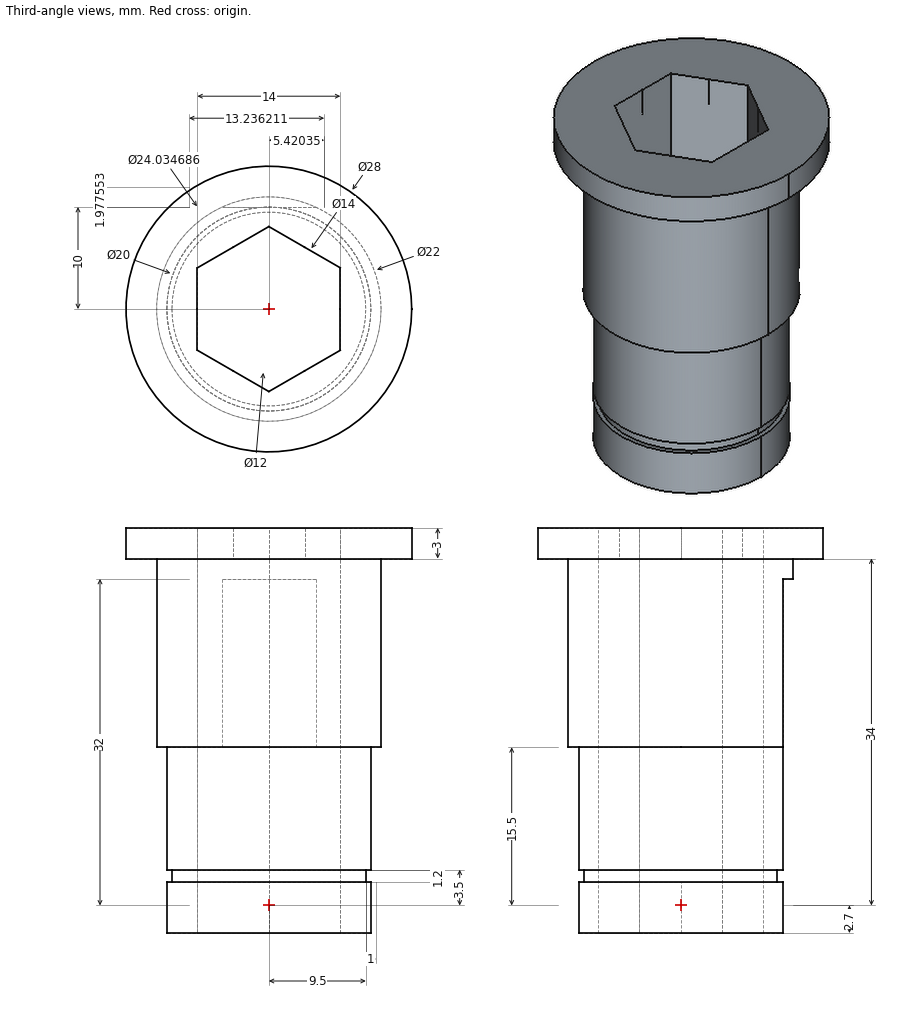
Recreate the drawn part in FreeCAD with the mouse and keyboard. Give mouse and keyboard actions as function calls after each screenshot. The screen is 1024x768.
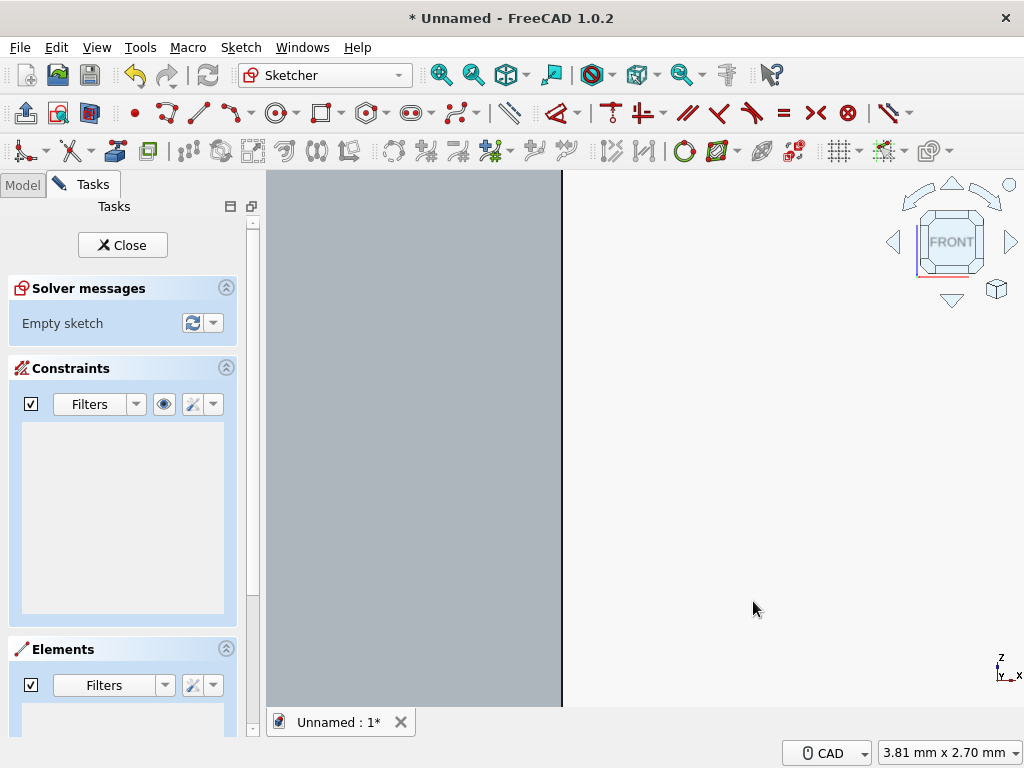
scroll(532, 402, up, 2)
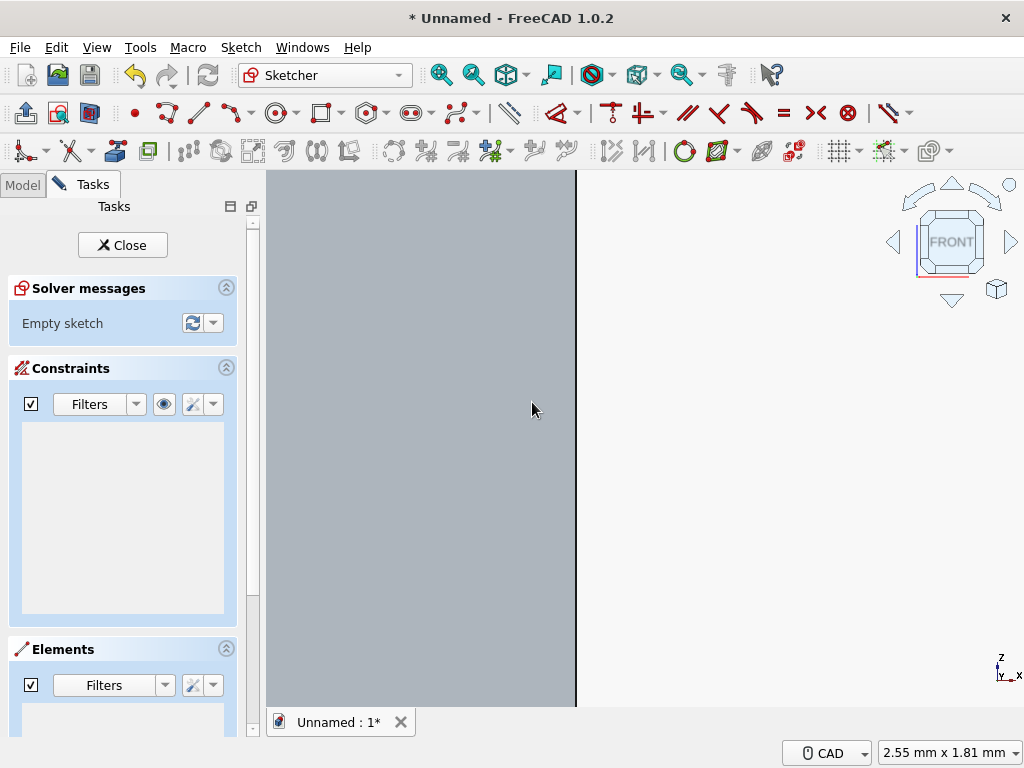
click(322, 114)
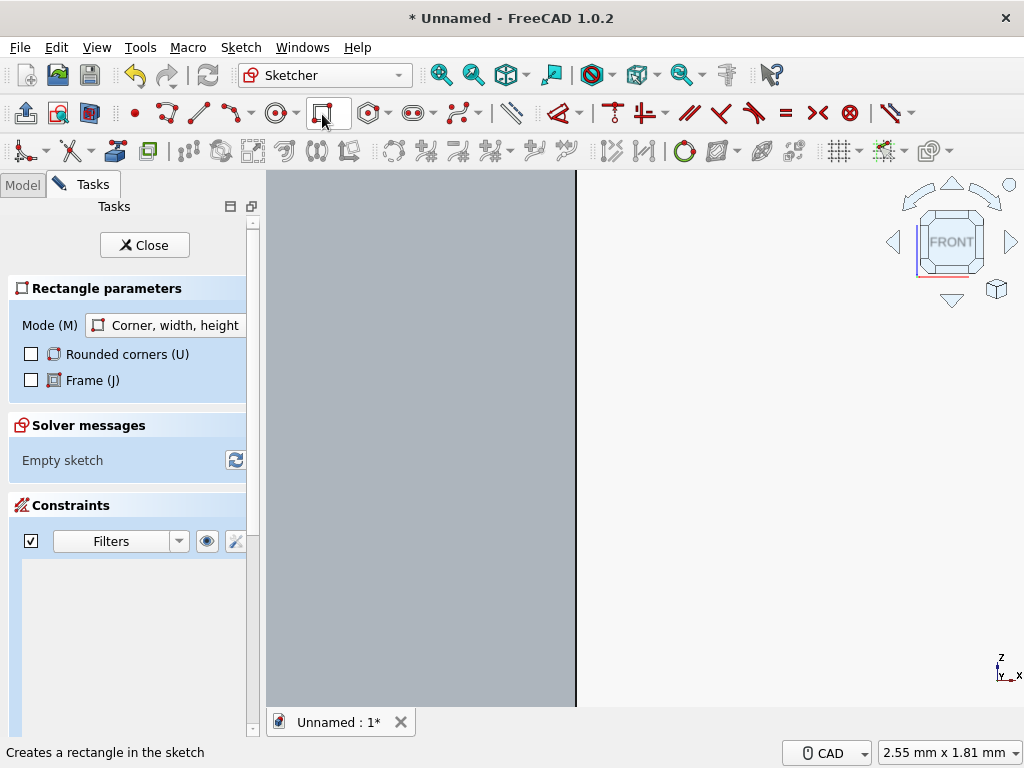
click(428, 260)
click(725, 617)
key(Escape)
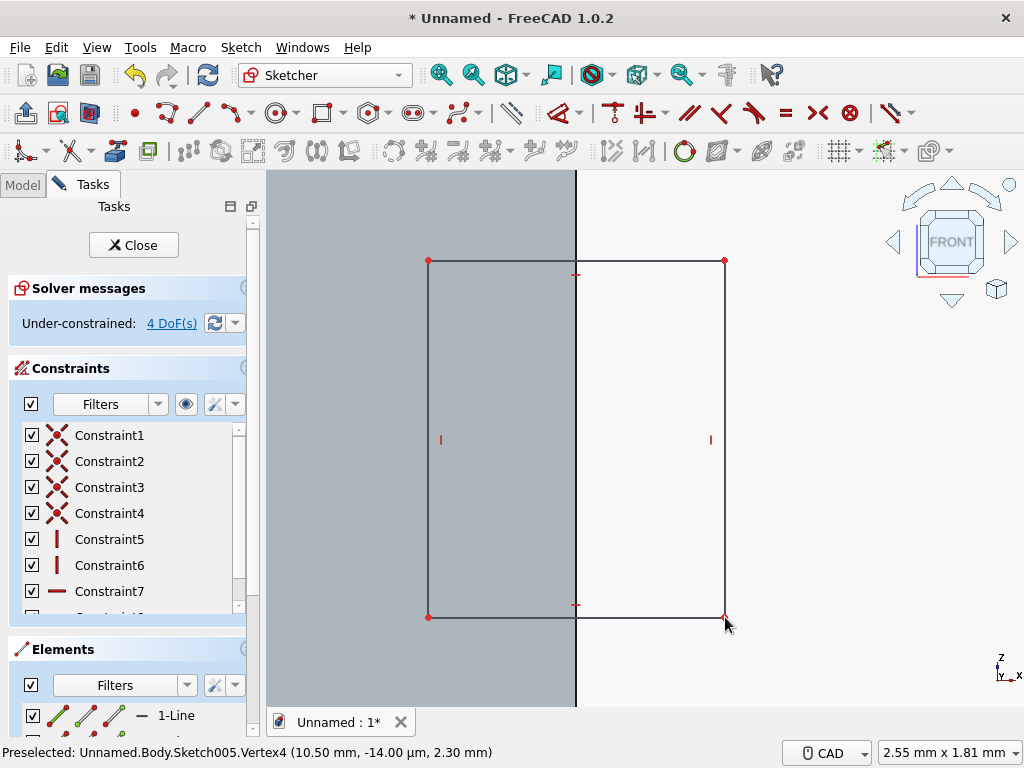
click(558, 114)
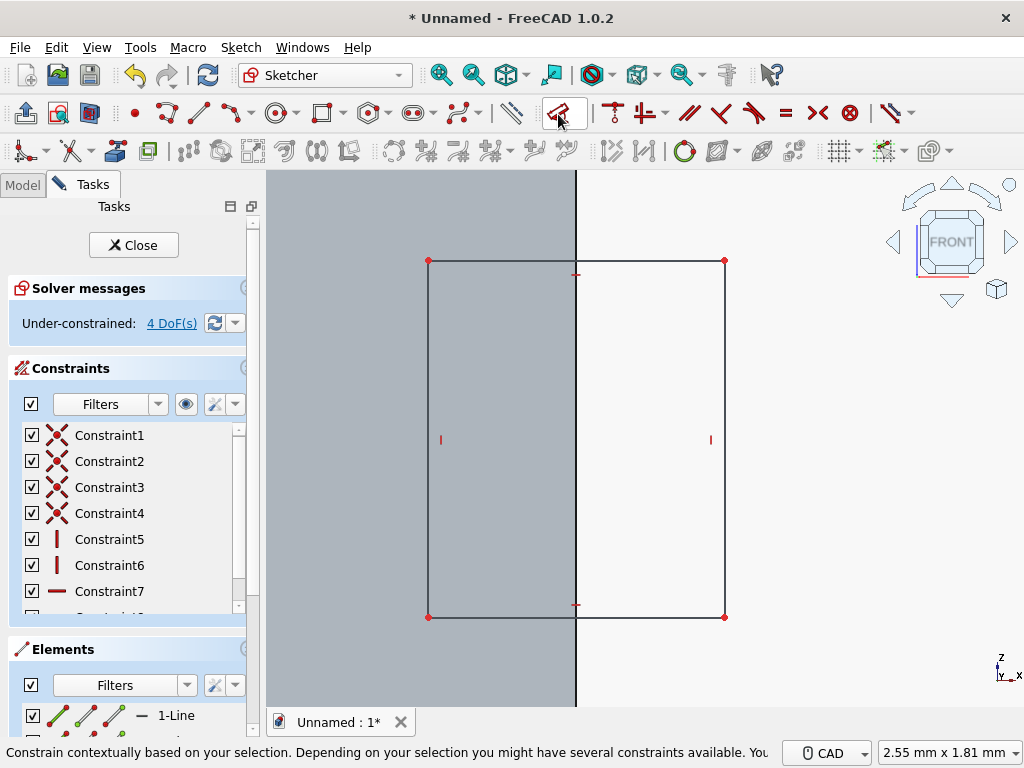
click(517, 618)
click(576, 652)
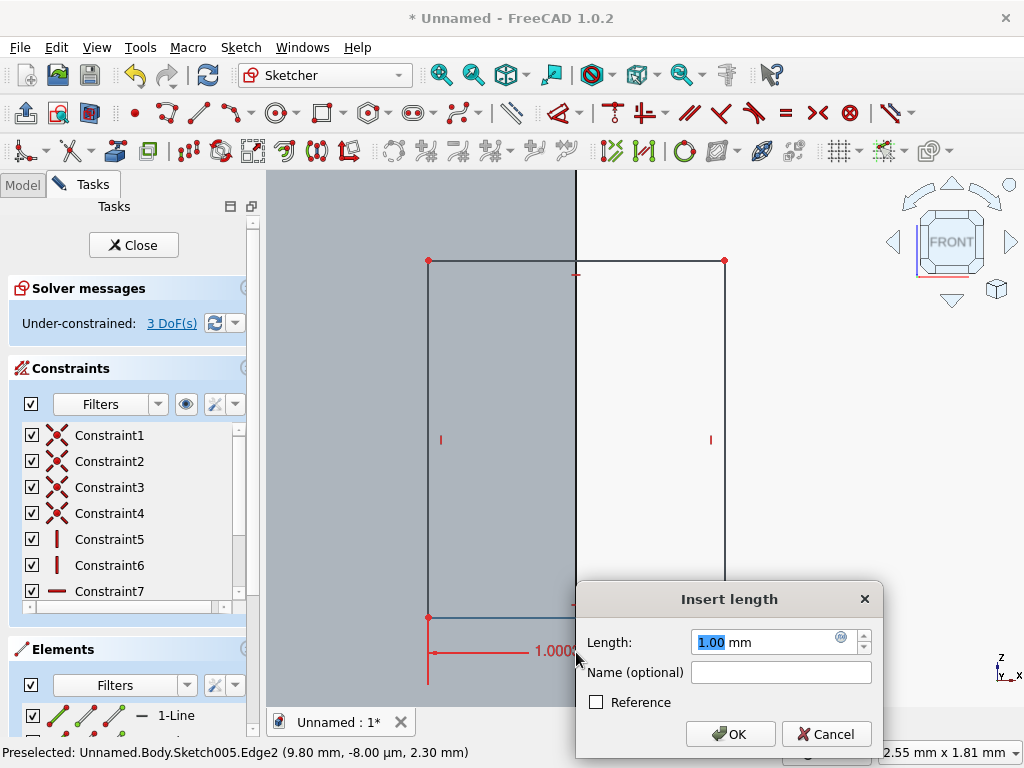
text(1)
key(Return)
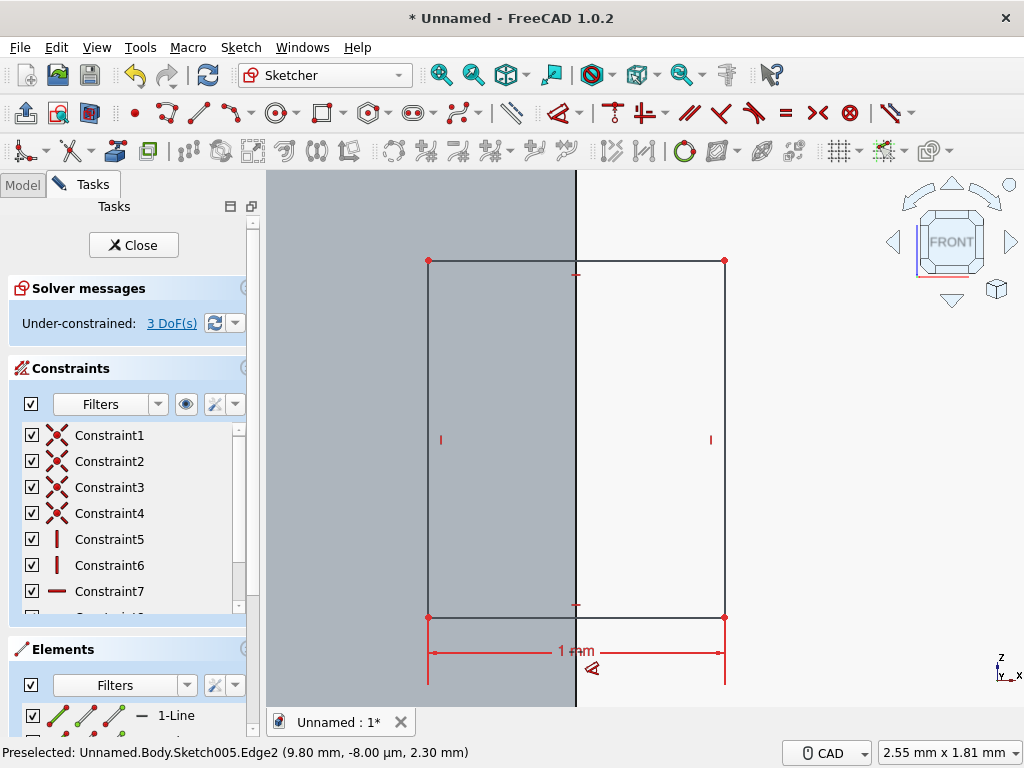
click(428, 368)
click(394, 440)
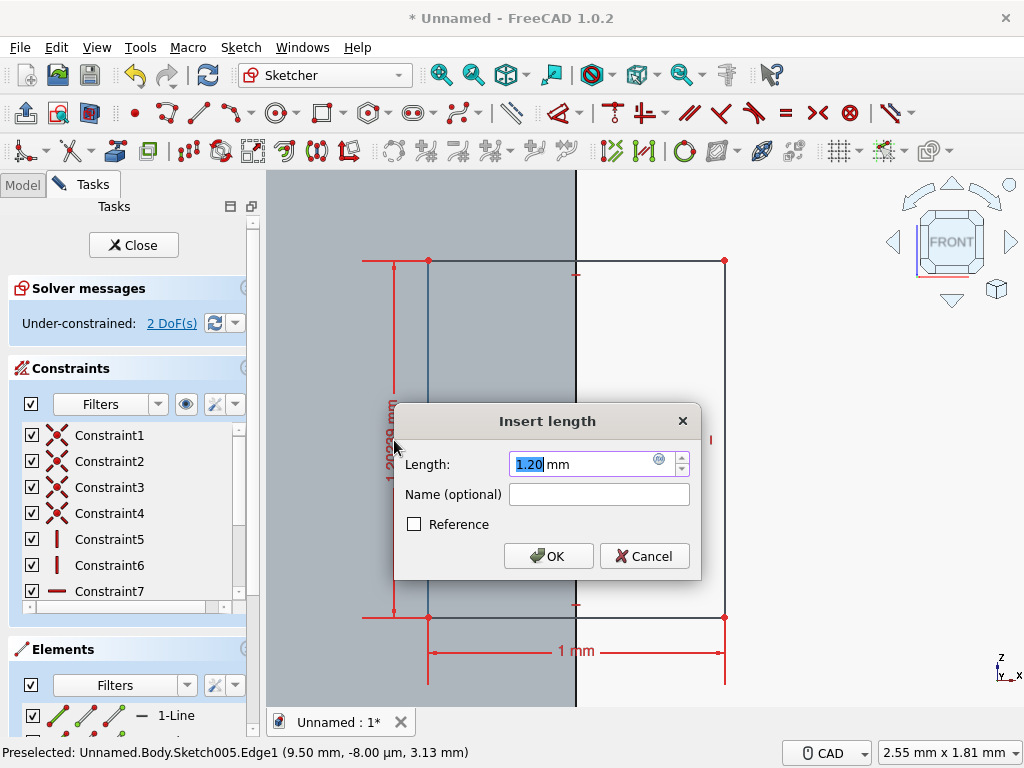
text(1.2)
key(Return)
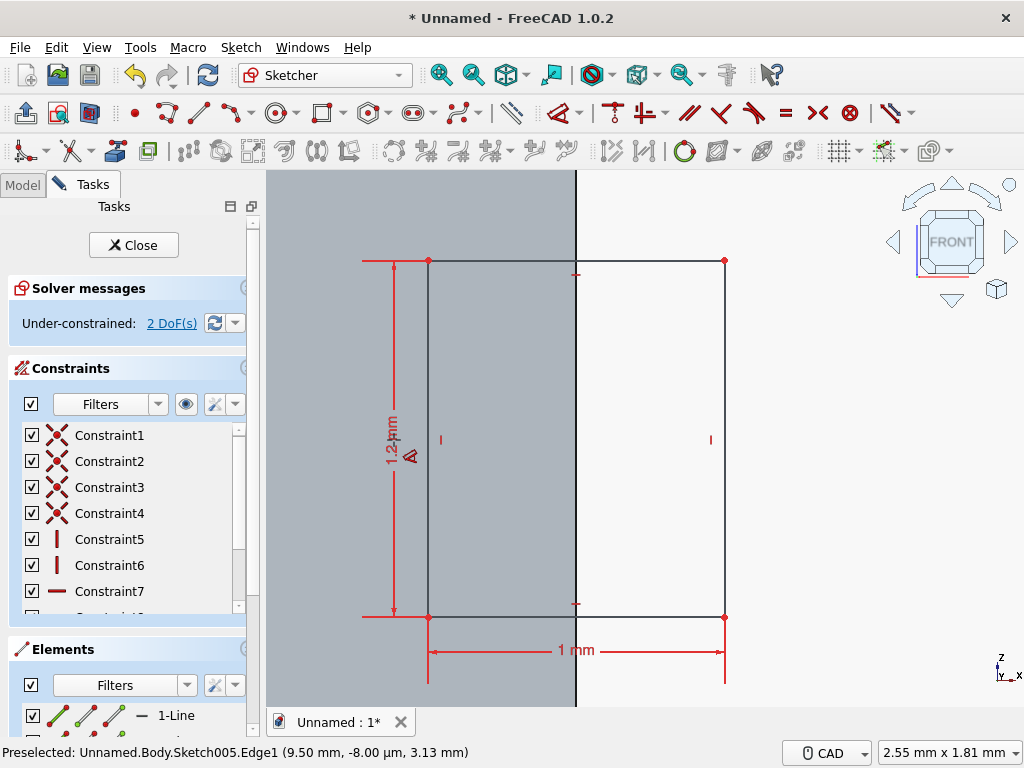
click(428, 261)
click(361, 227)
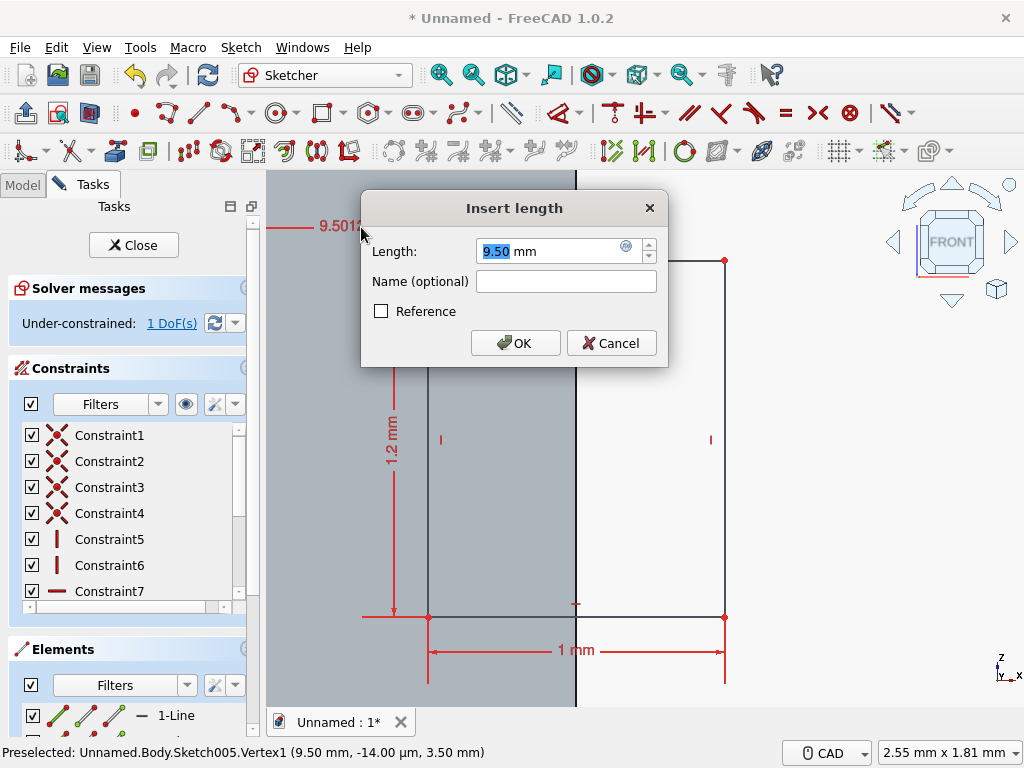
text(9.5)
key(Return)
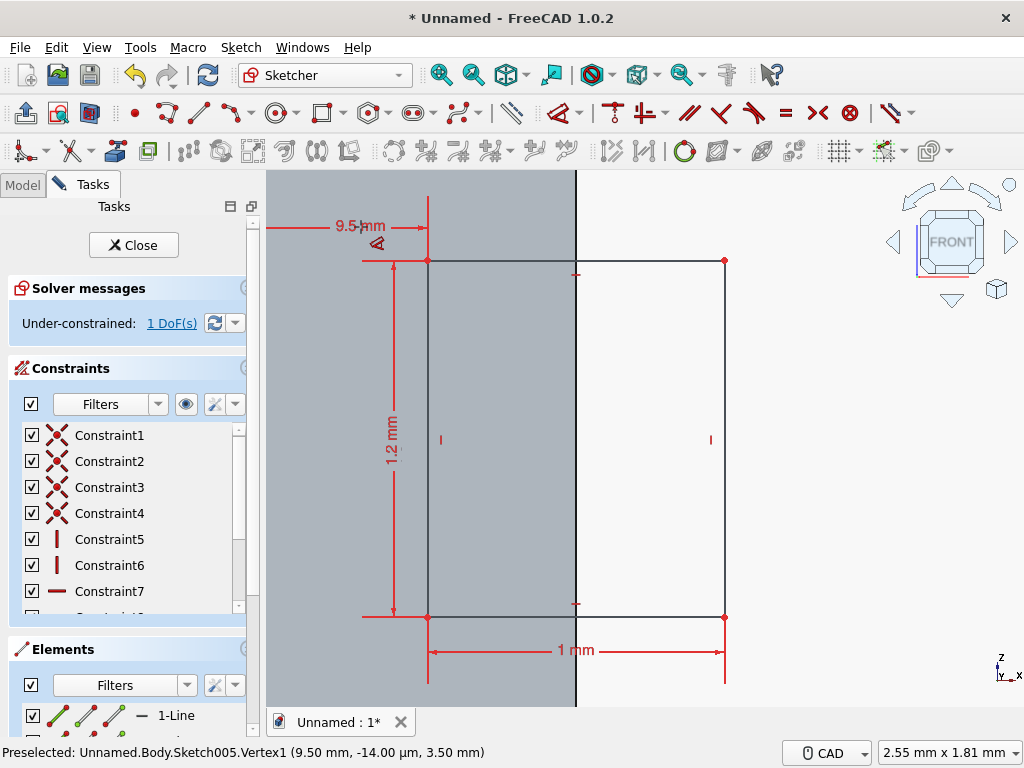
click(428, 261)
click(462, 470)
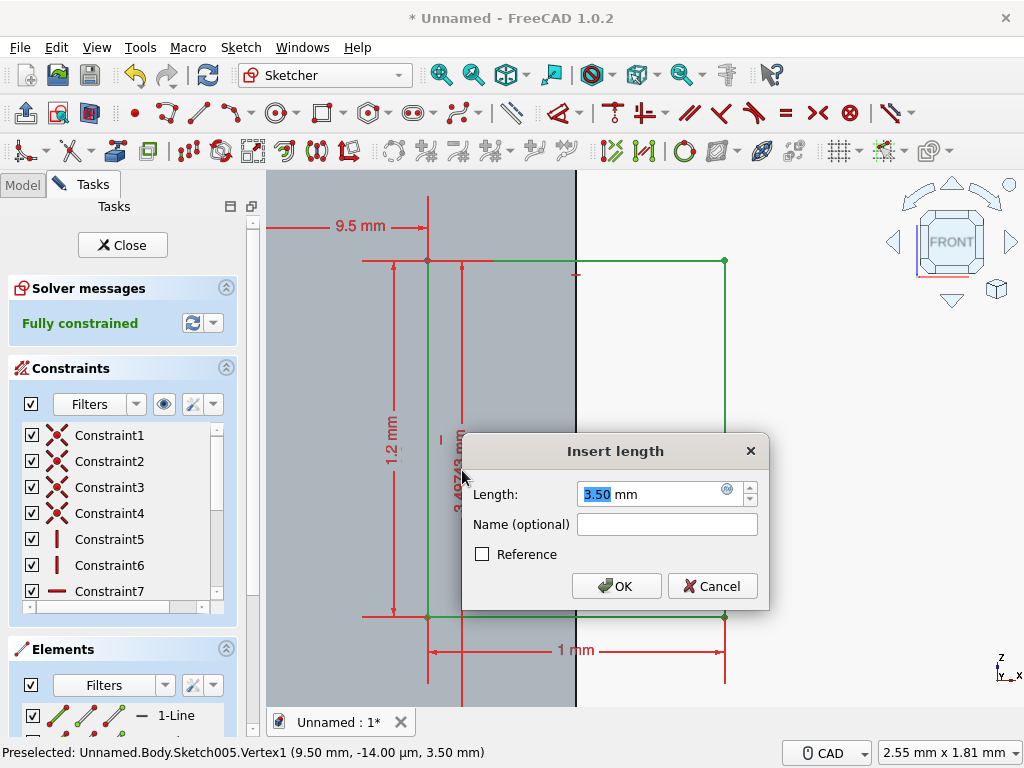
text(3.5)
key(Return)
key(Escape)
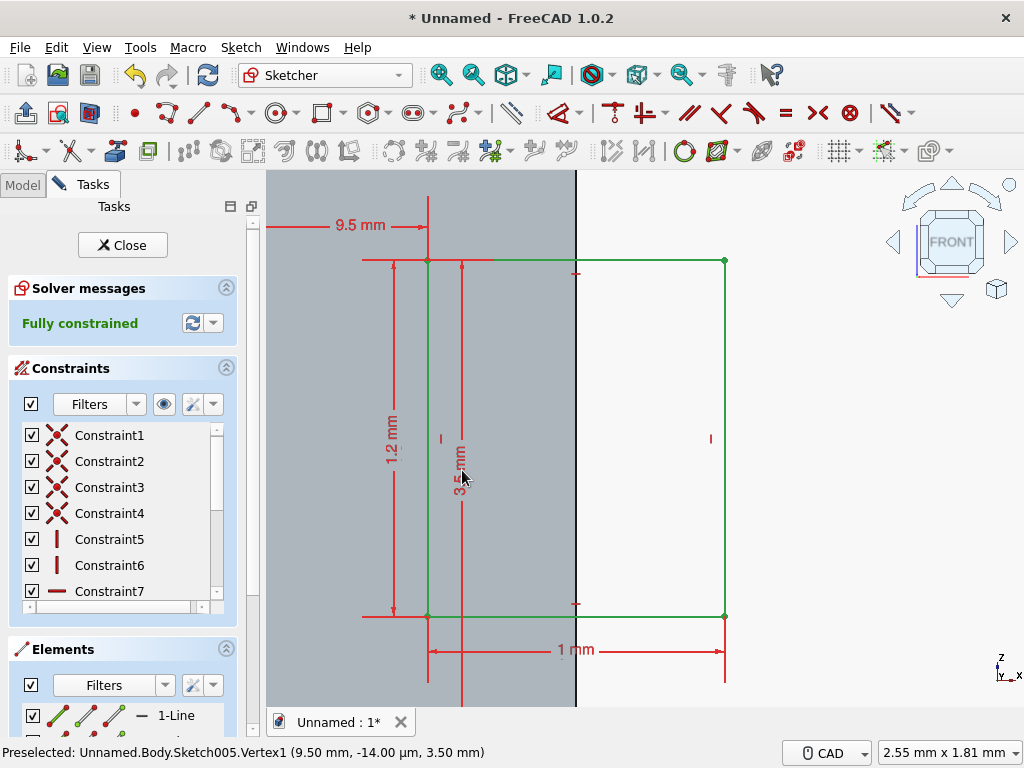
click(123, 245)